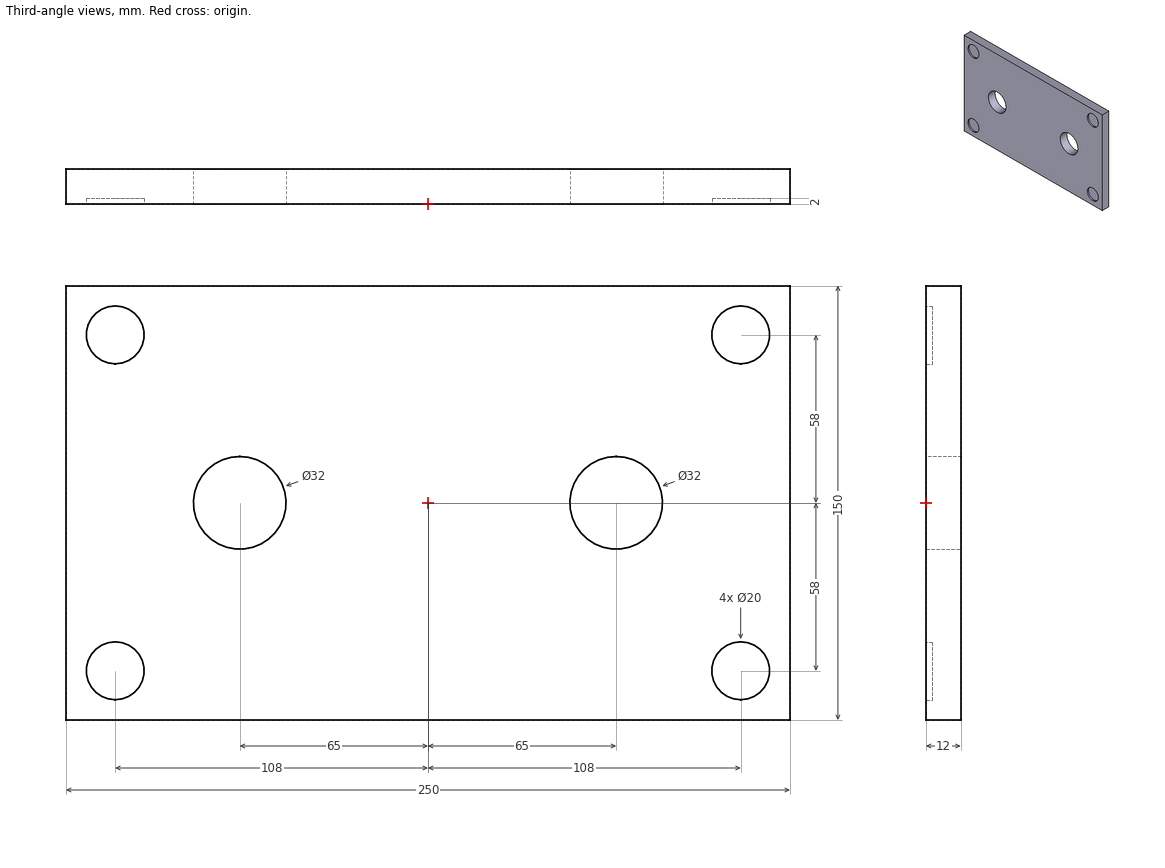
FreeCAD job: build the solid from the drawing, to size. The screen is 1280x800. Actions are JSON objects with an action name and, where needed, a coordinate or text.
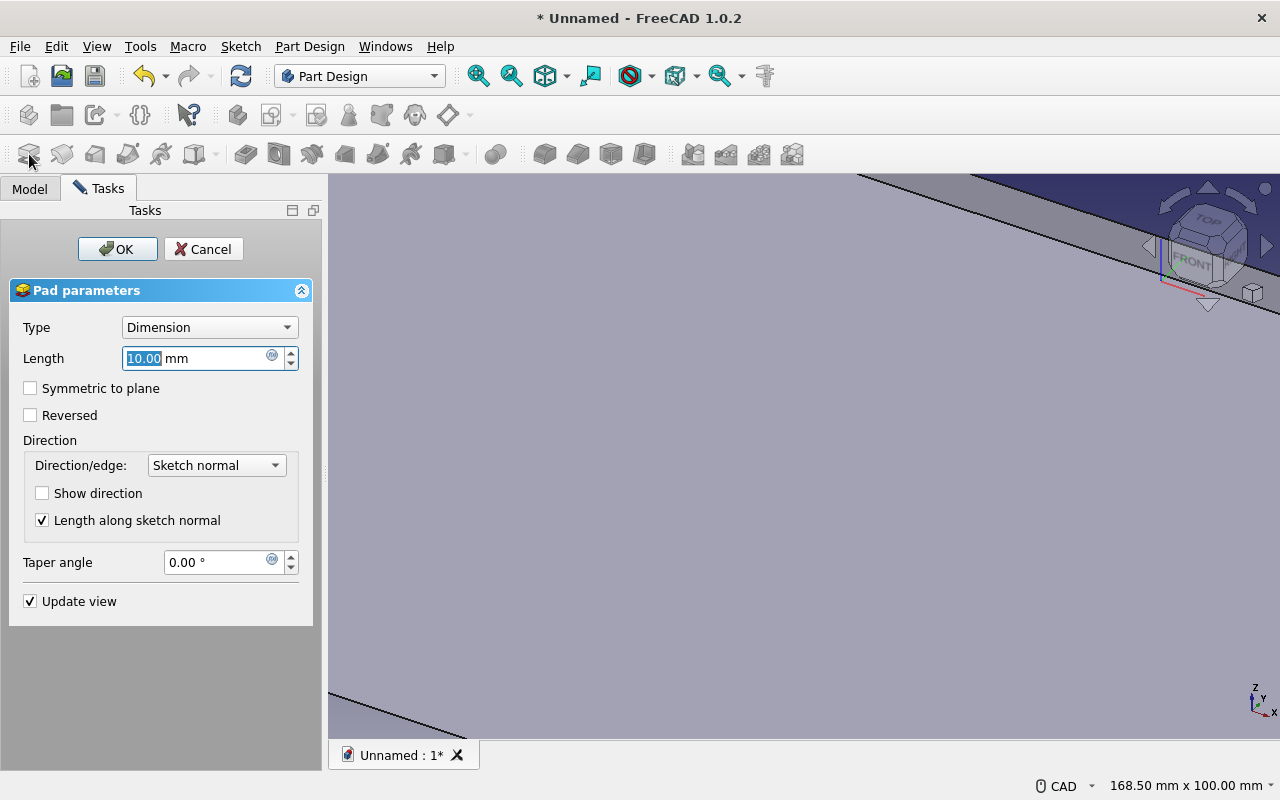
{"action": "type", "text": "12"}
{"action": "key", "text": "Tab"}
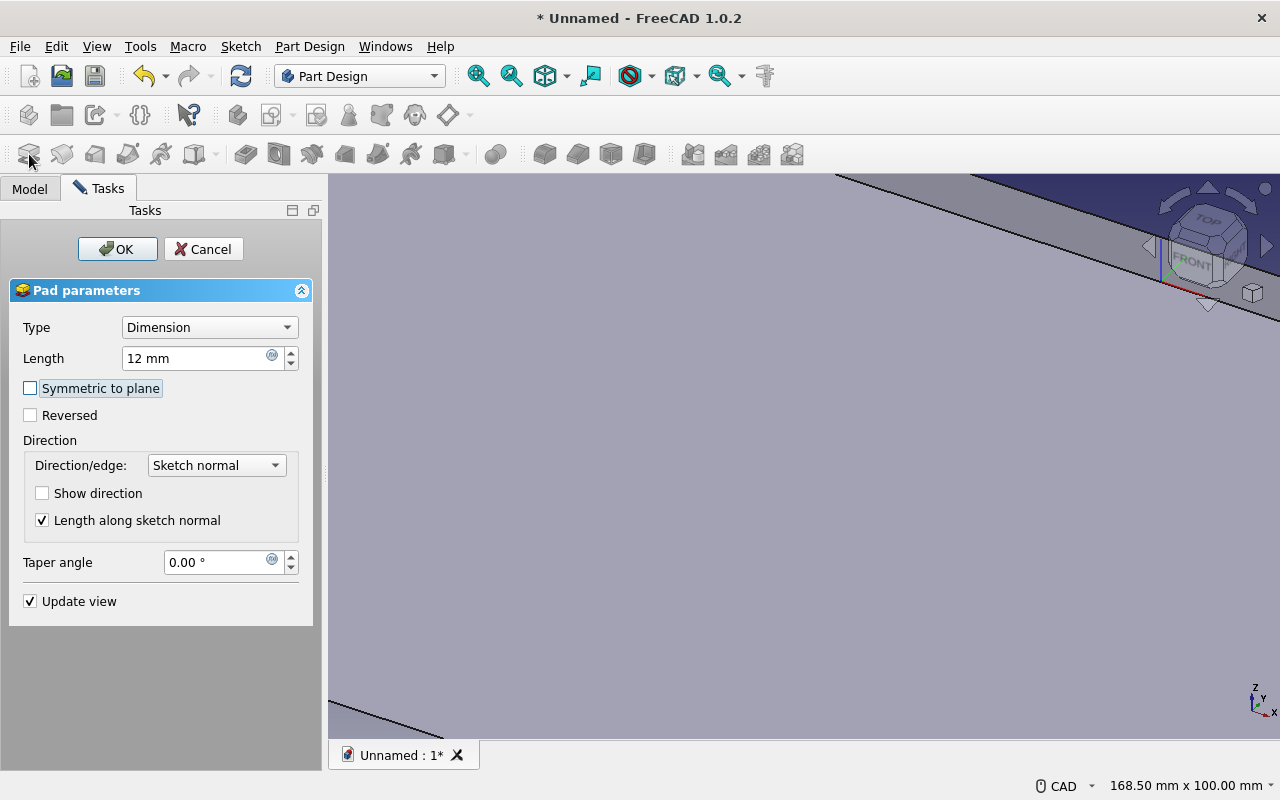
{"action": "left_click", "coordinate": [31, 415]}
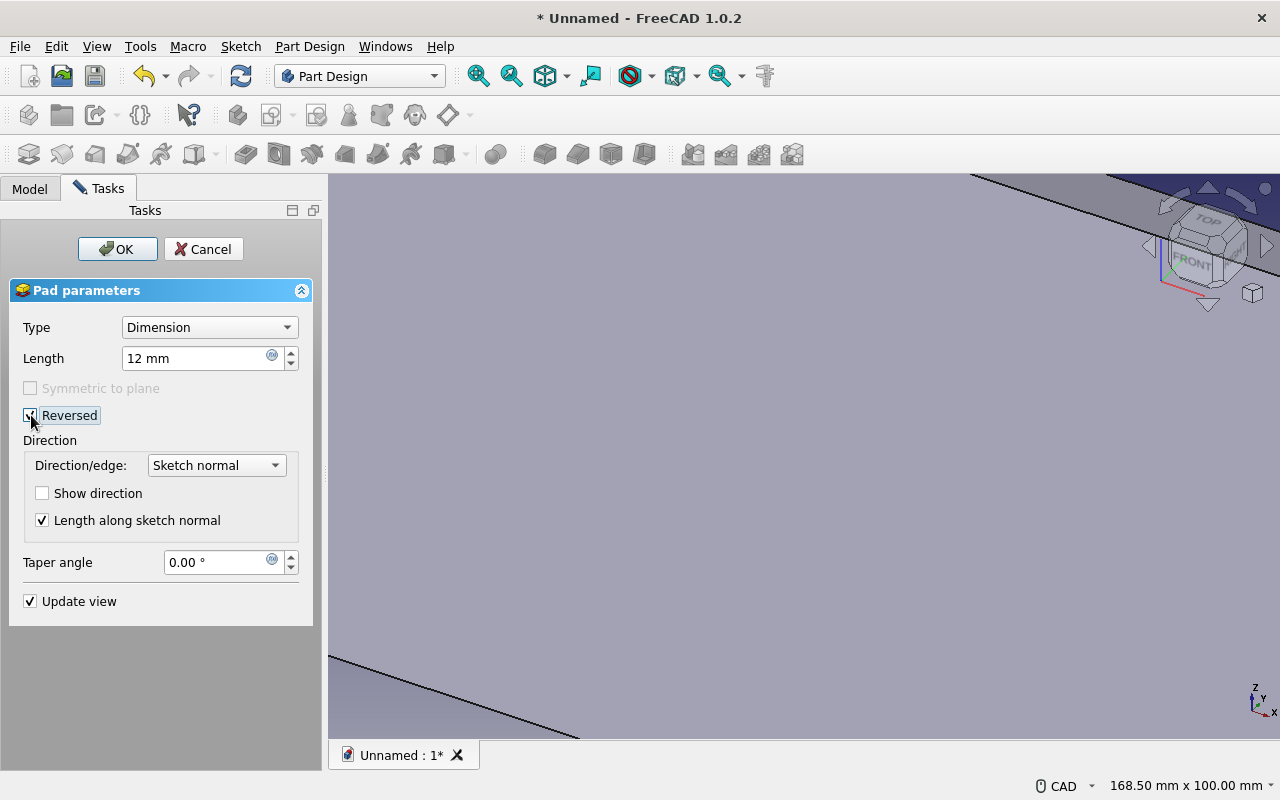
{"action": "left_click", "coordinate": [118, 249]}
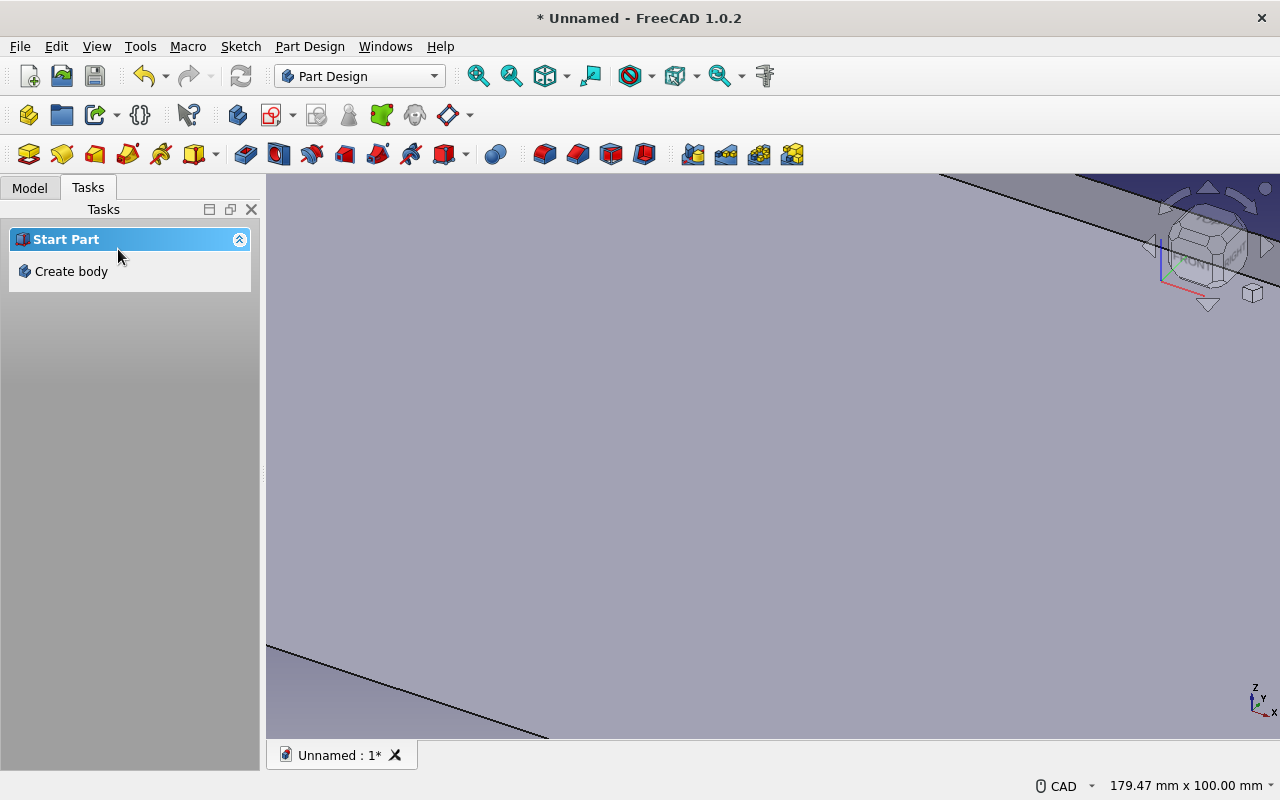
{"action": "left_click", "coordinate": [479, 76]}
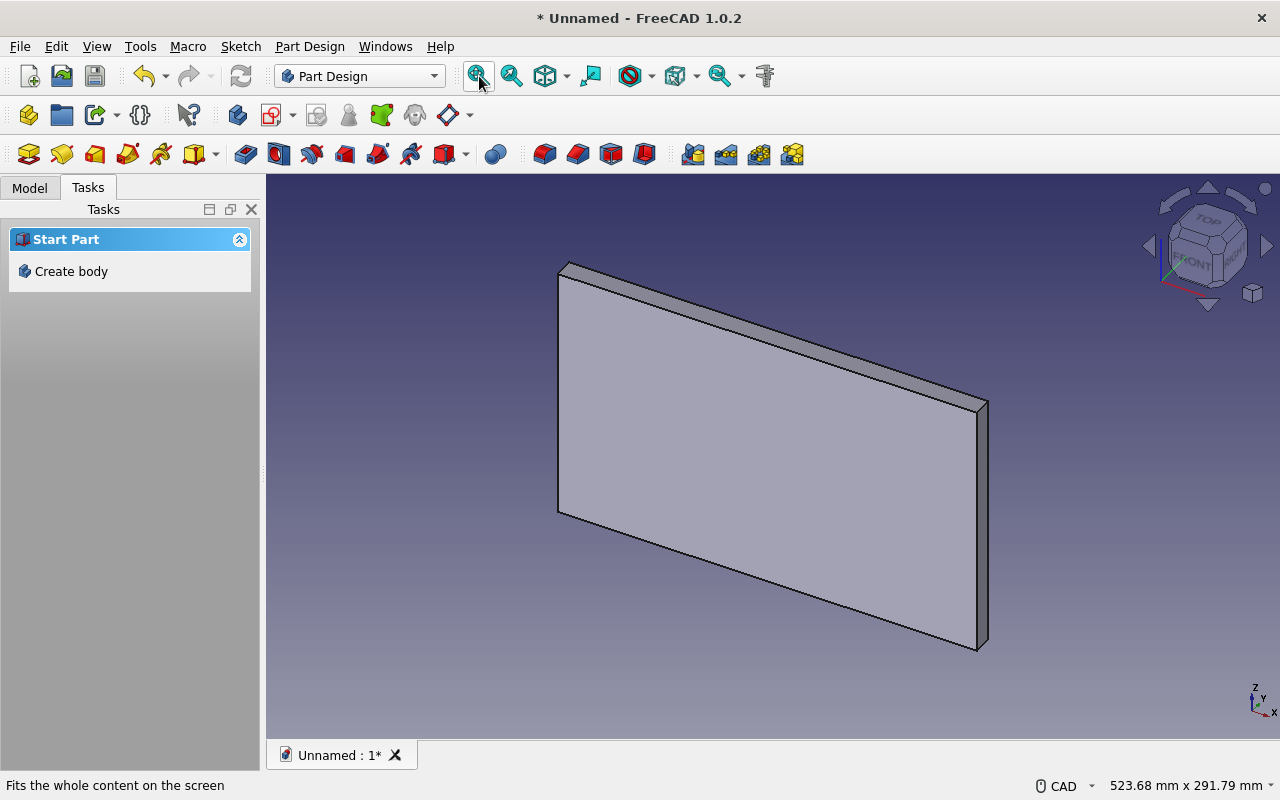
{"action": "left_click", "coordinate": [270, 116]}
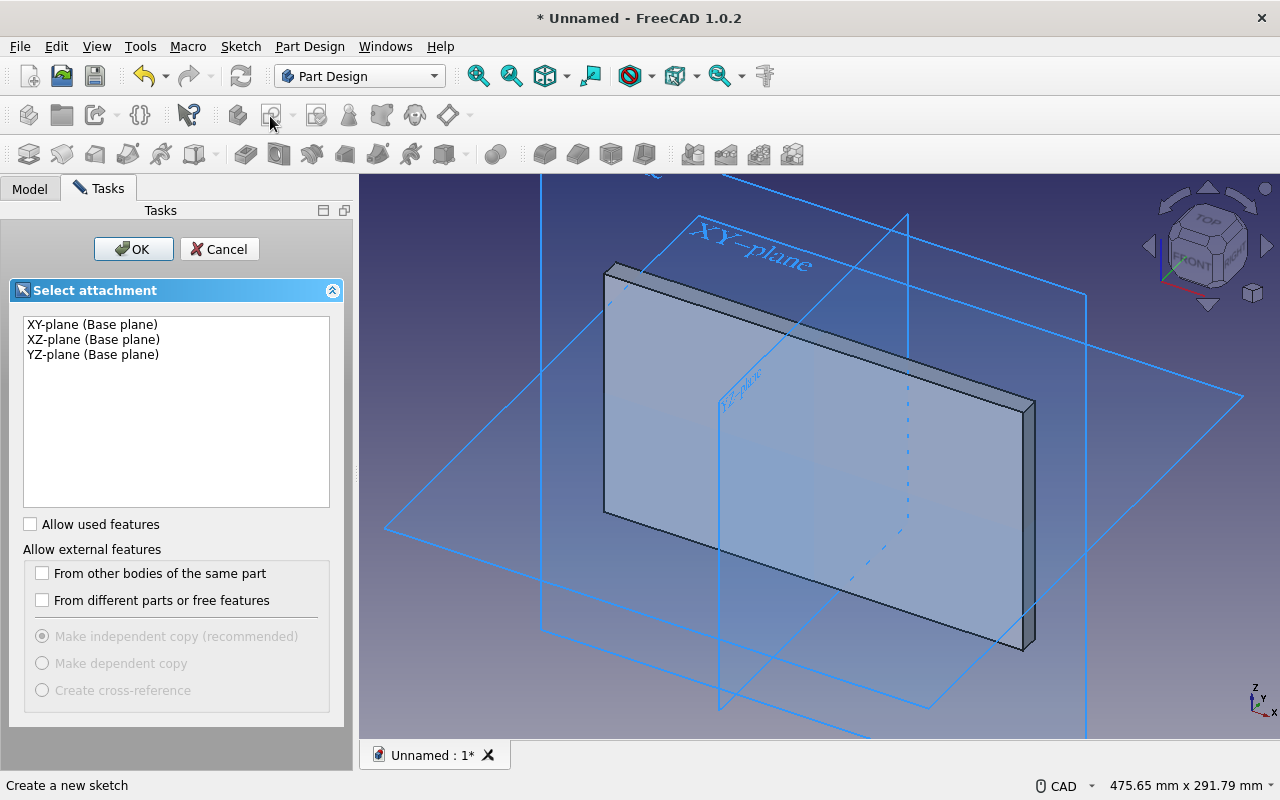
{"action": "left_click", "coordinate": [84, 340]}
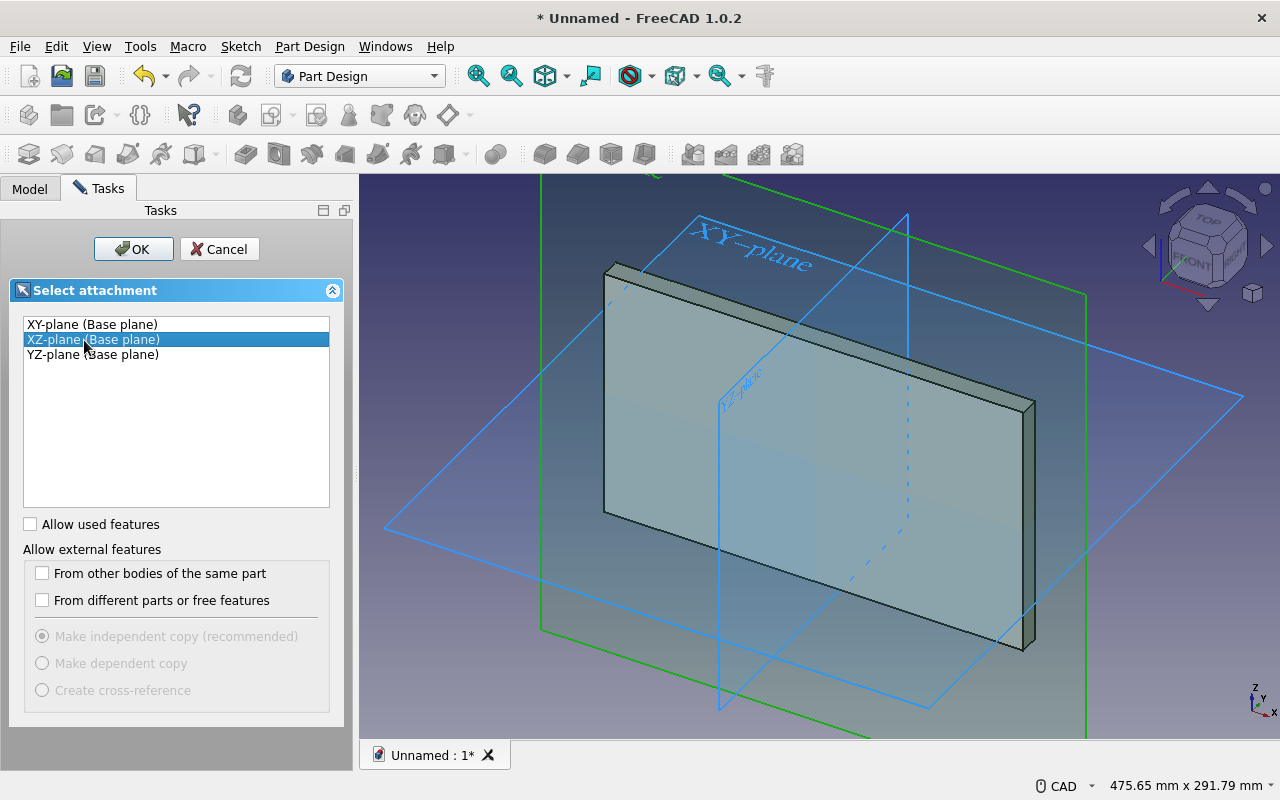
{"action": "left_click", "coordinate": [134, 249]}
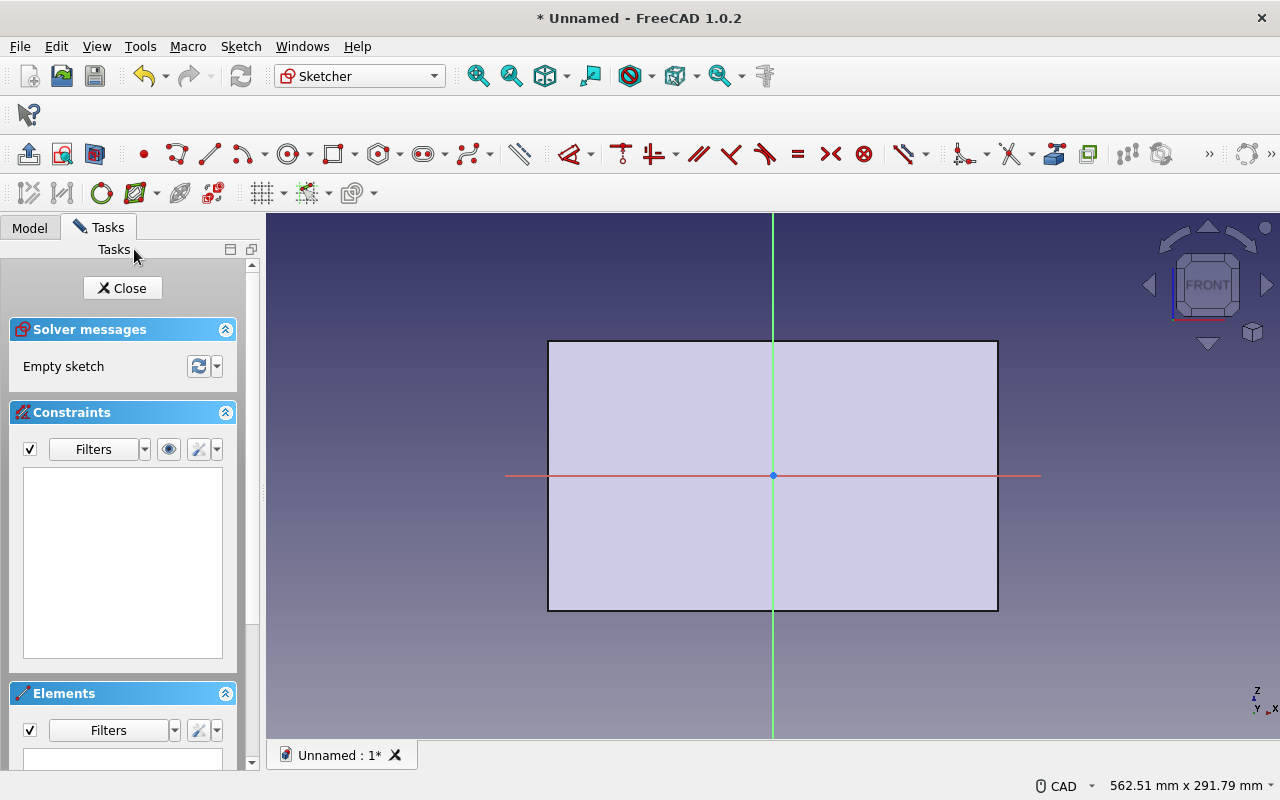
{"action": "scroll", "coordinate": [912, 476], "scroll_direction": "up", "scroll_amount": 2}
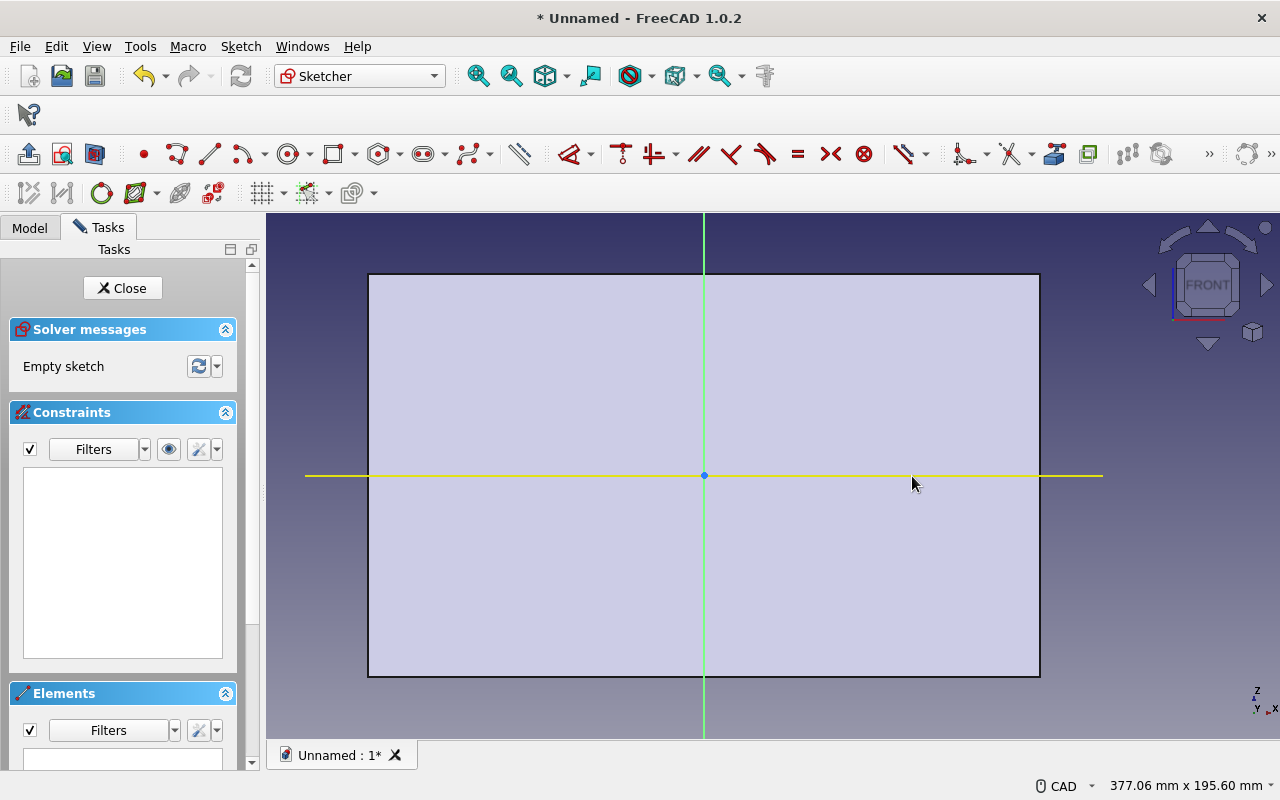
{"action": "left_click", "coordinate": [288, 154]}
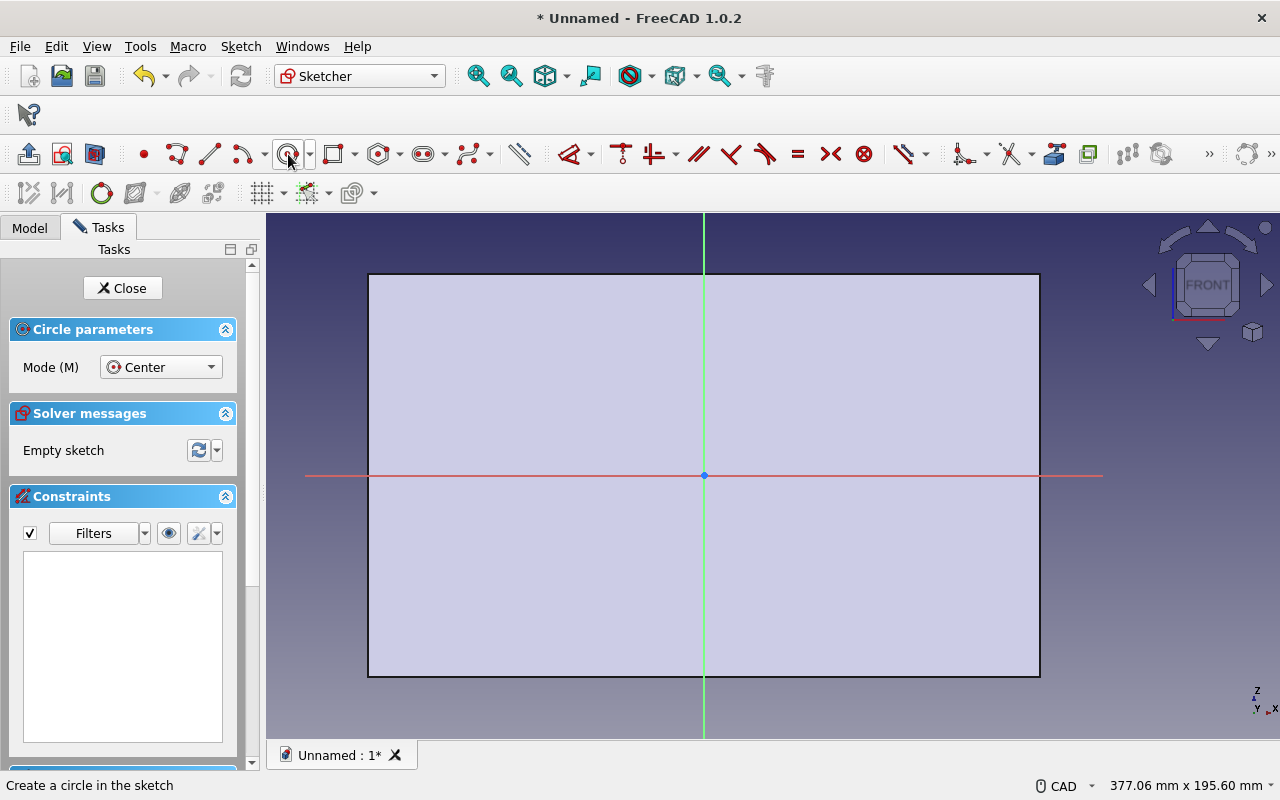
{"action": "left_click", "coordinate": [995, 632]}
{"action": "mouse_move", "coordinate": [1014, 613]}